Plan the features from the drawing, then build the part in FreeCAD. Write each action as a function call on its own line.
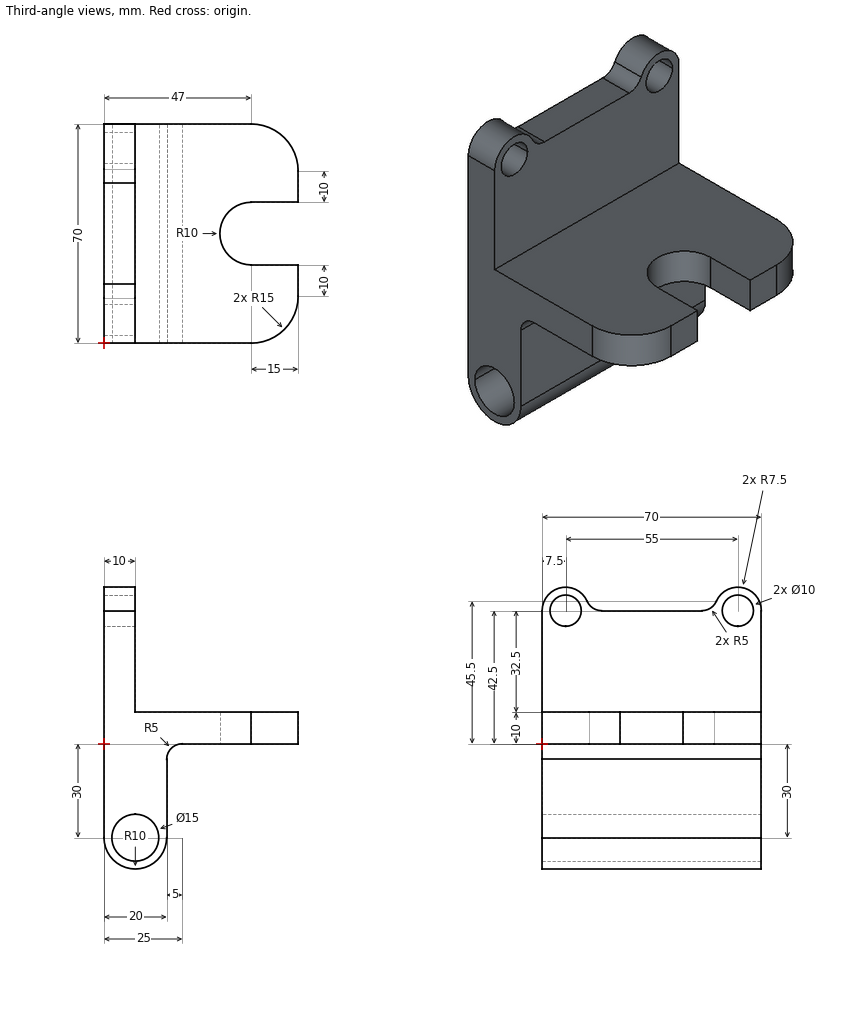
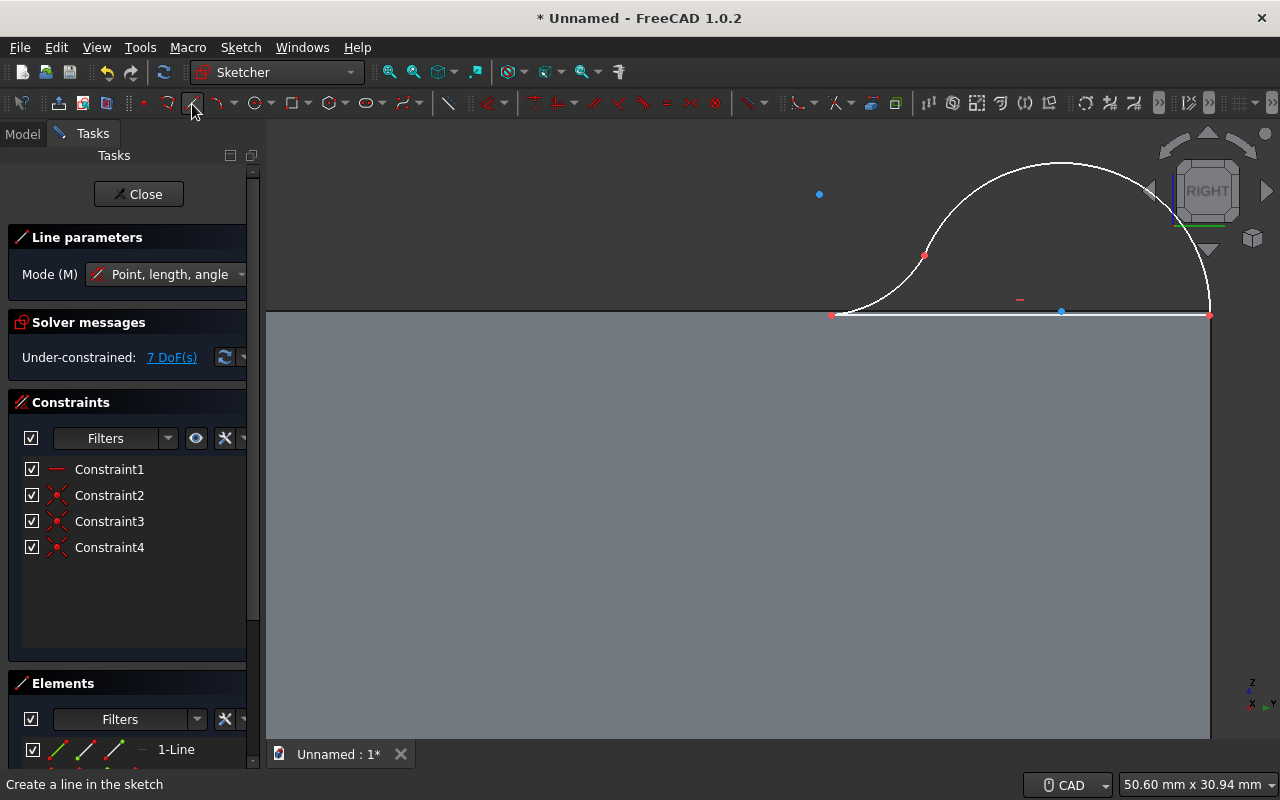
scroll(818, 293, down, 5)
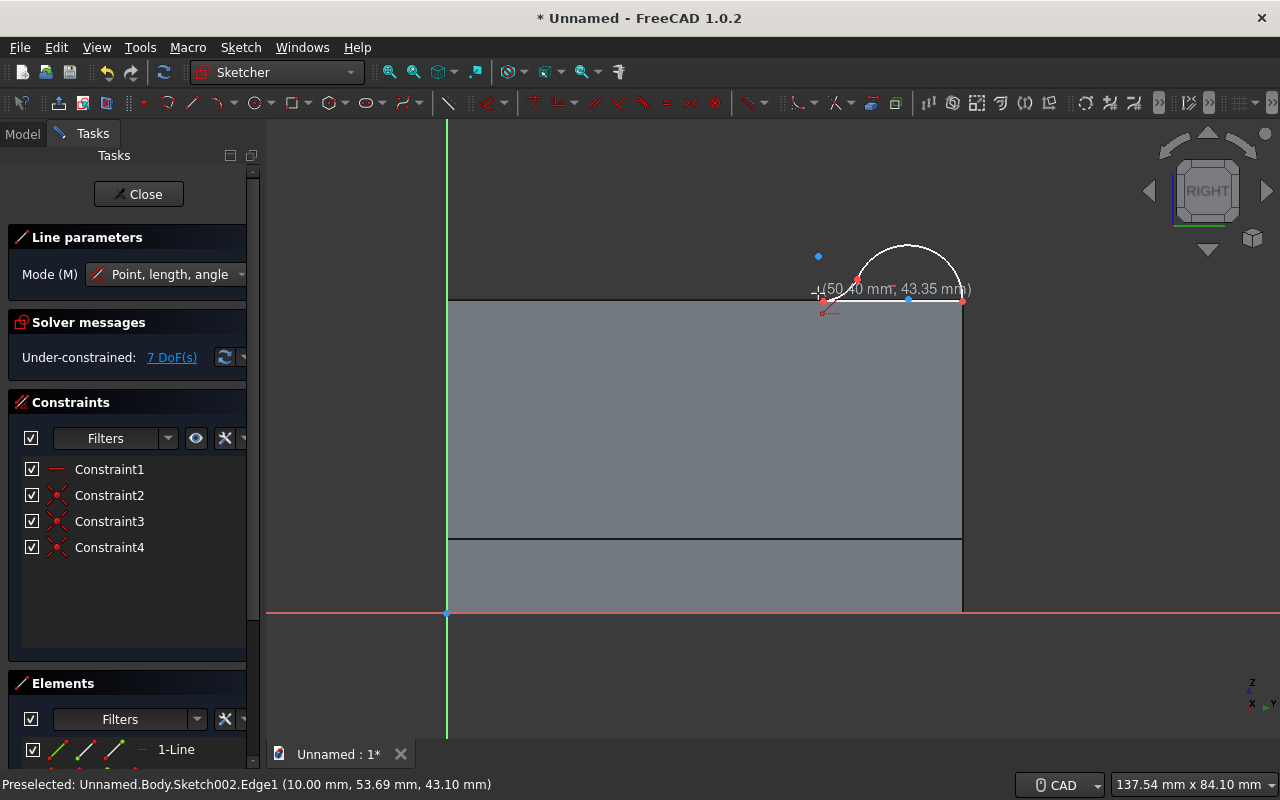
click(447, 300)
click(587, 300)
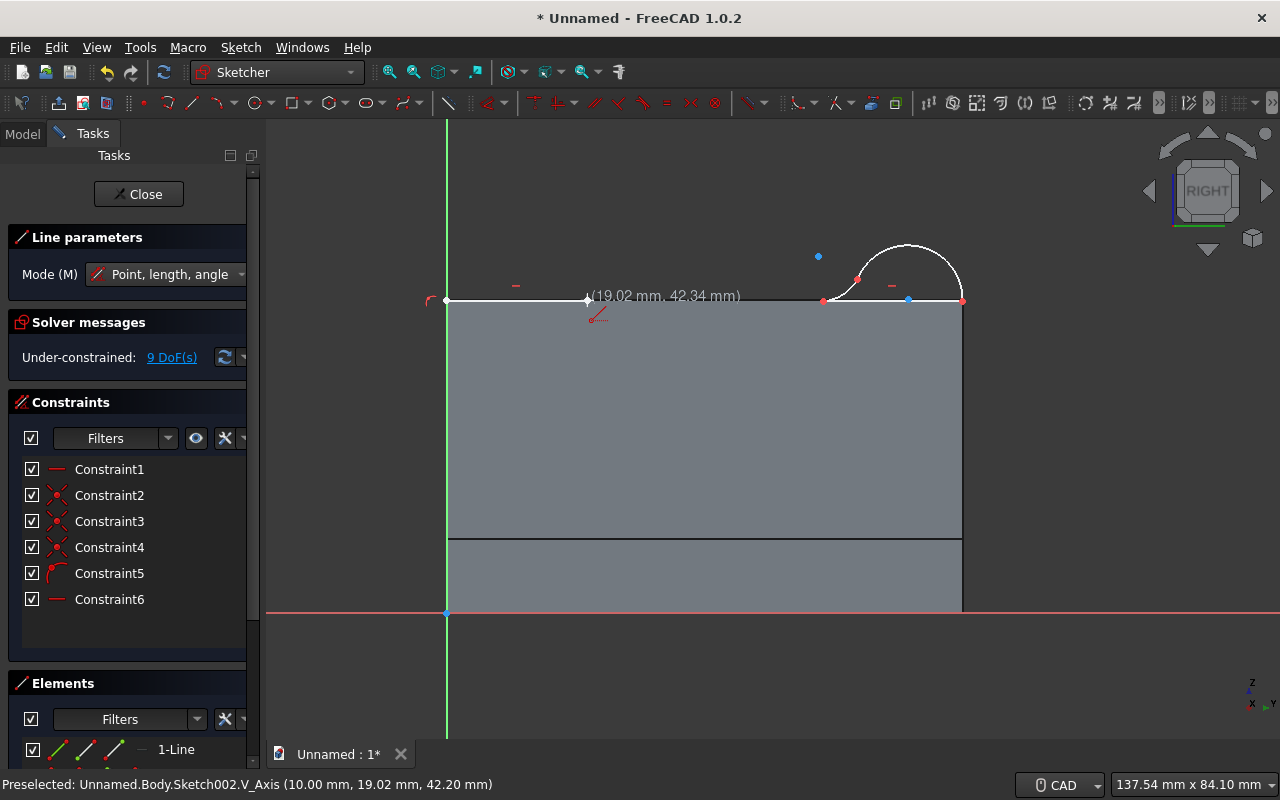
click(218, 104)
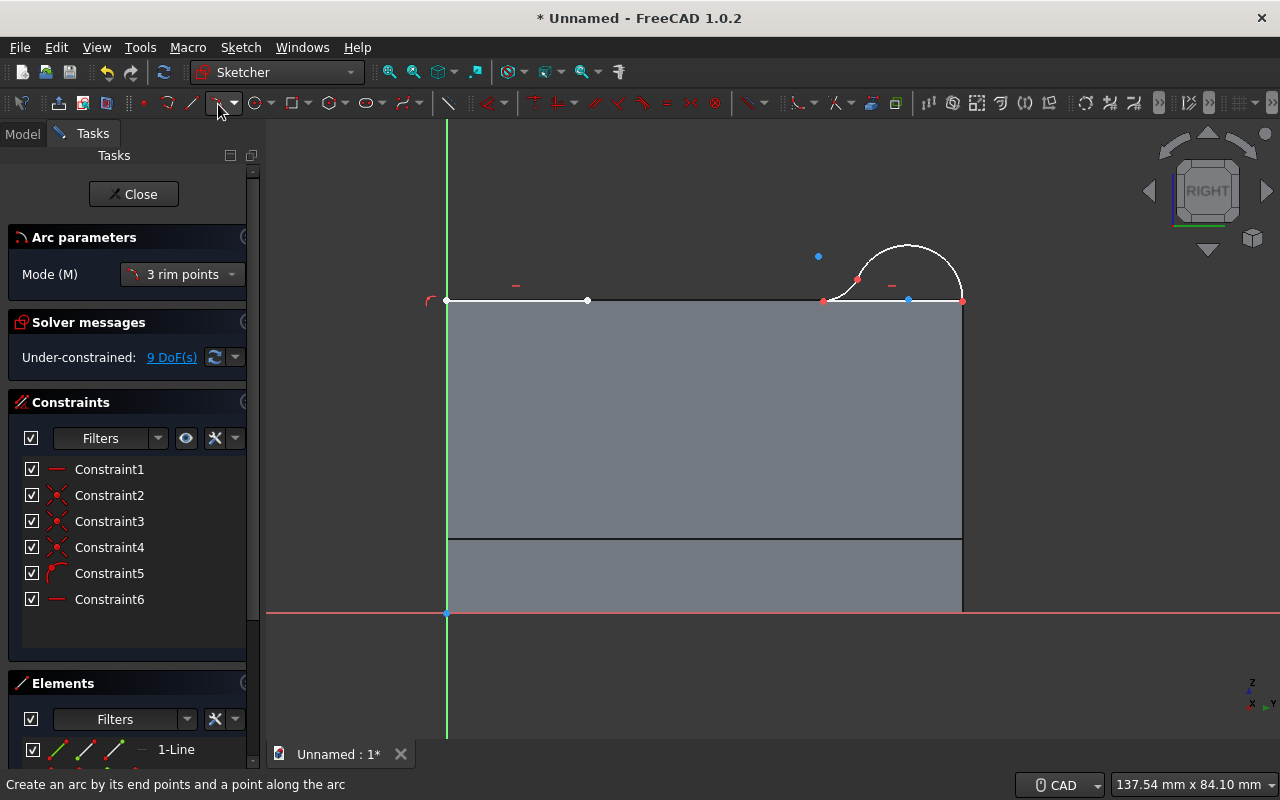
click(587, 301)
click(553, 278)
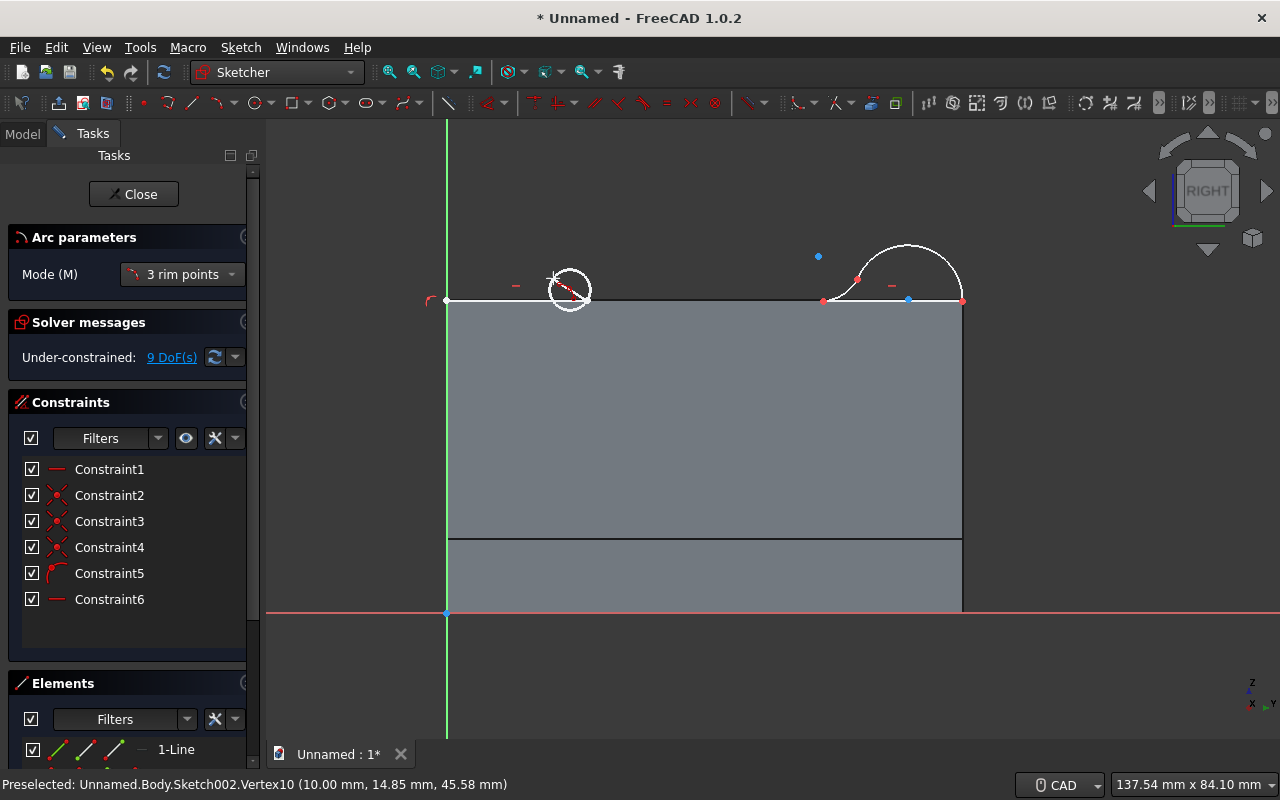
scroll(566, 294, up, 5)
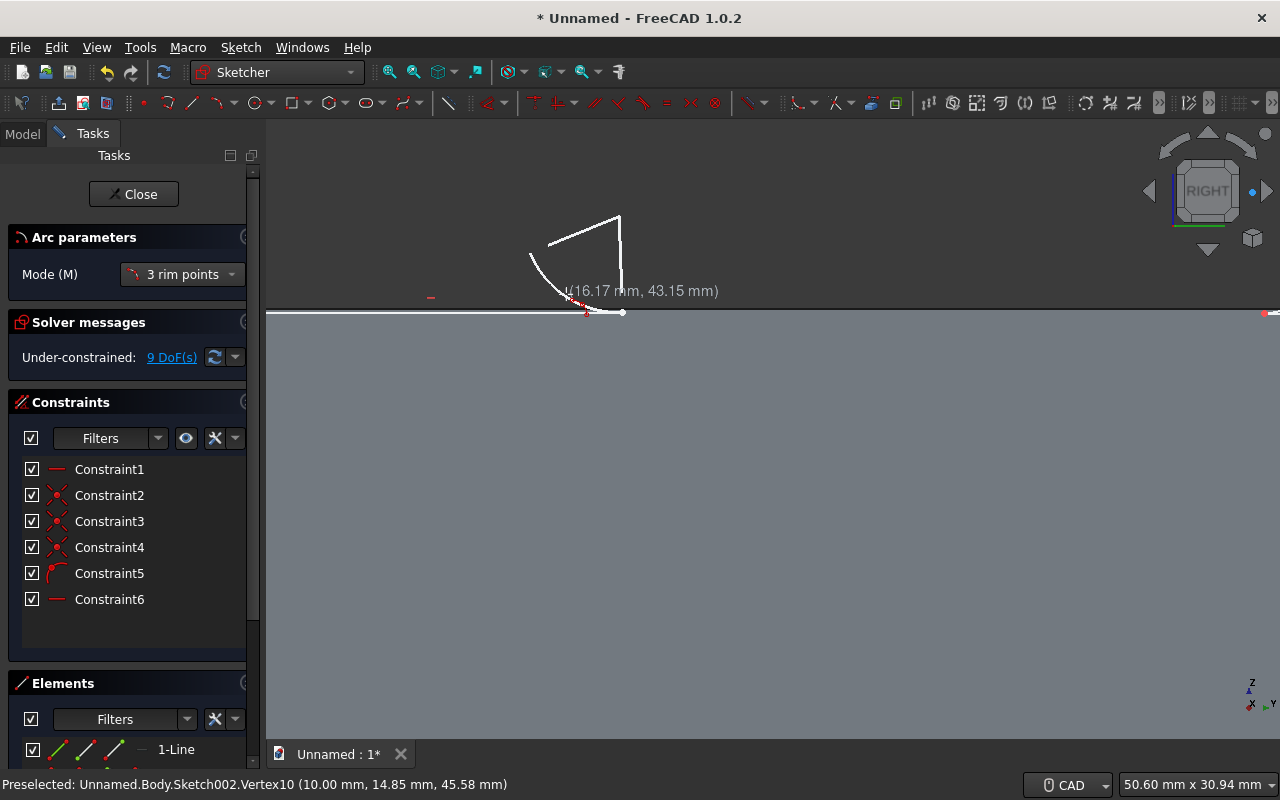
click(566, 293)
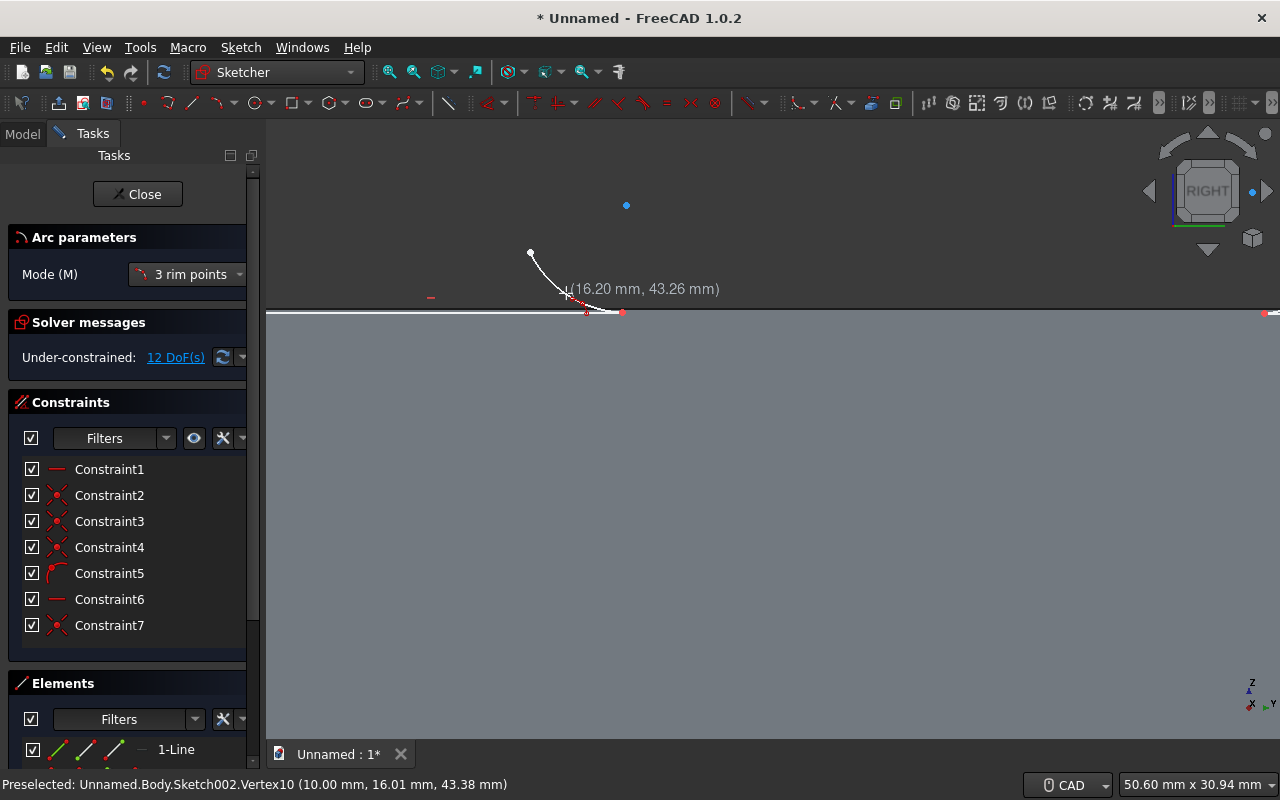
click(530, 253)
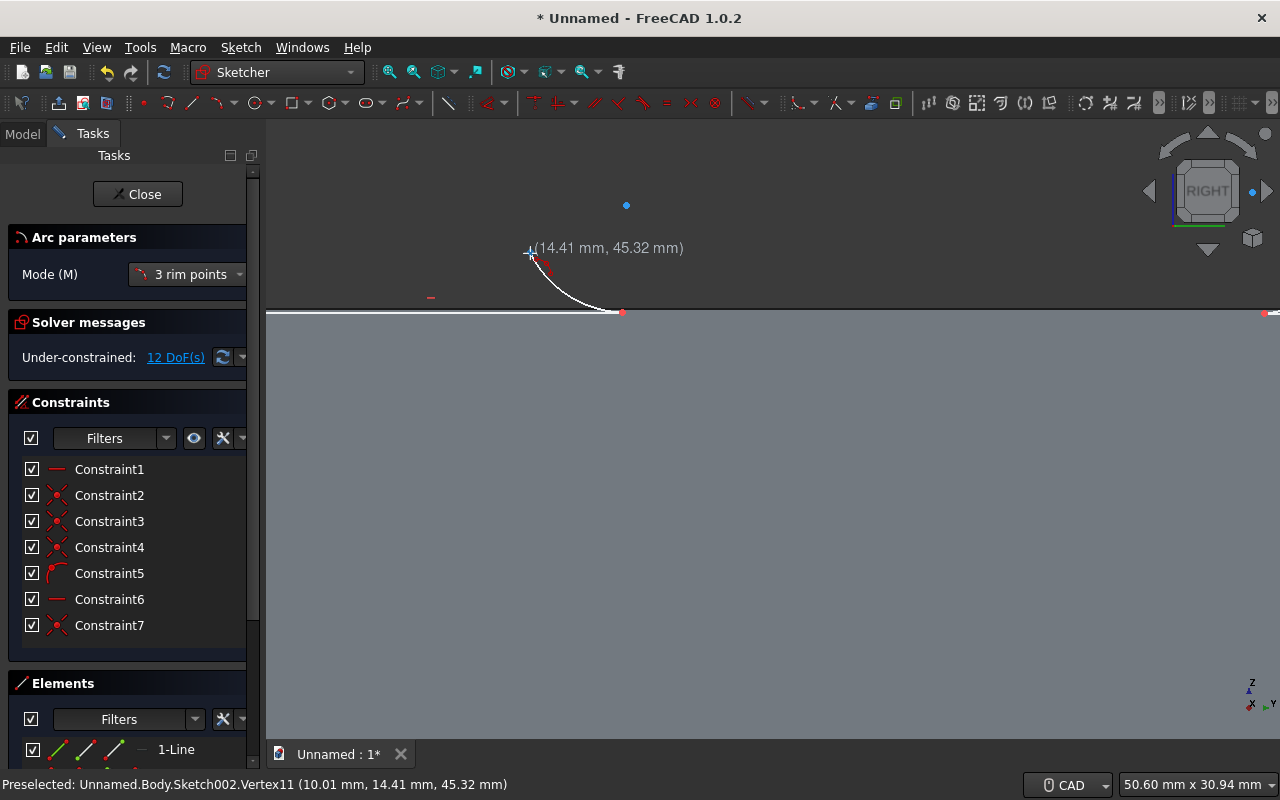
scroll(566, 294, down, 5)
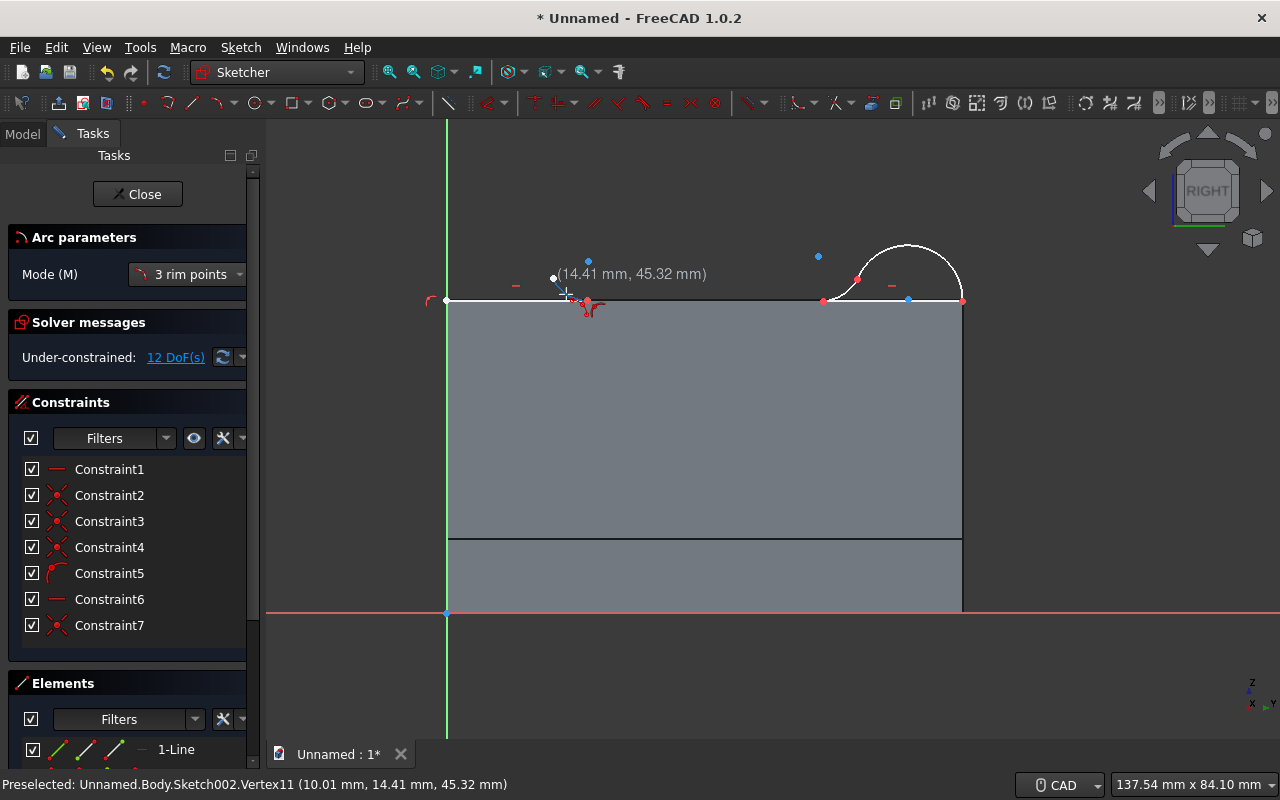
click(447, 301)
click(491, 246)
key(Escape)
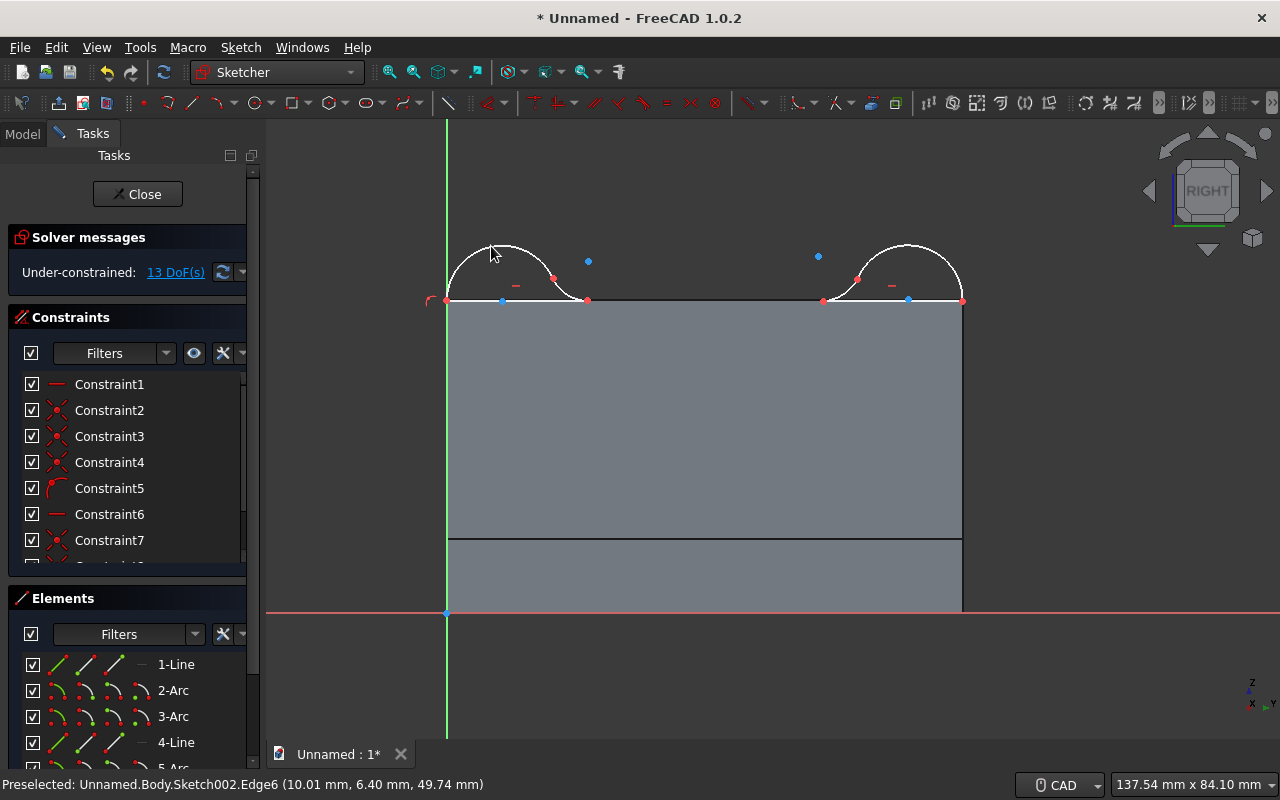
click(865, 301)